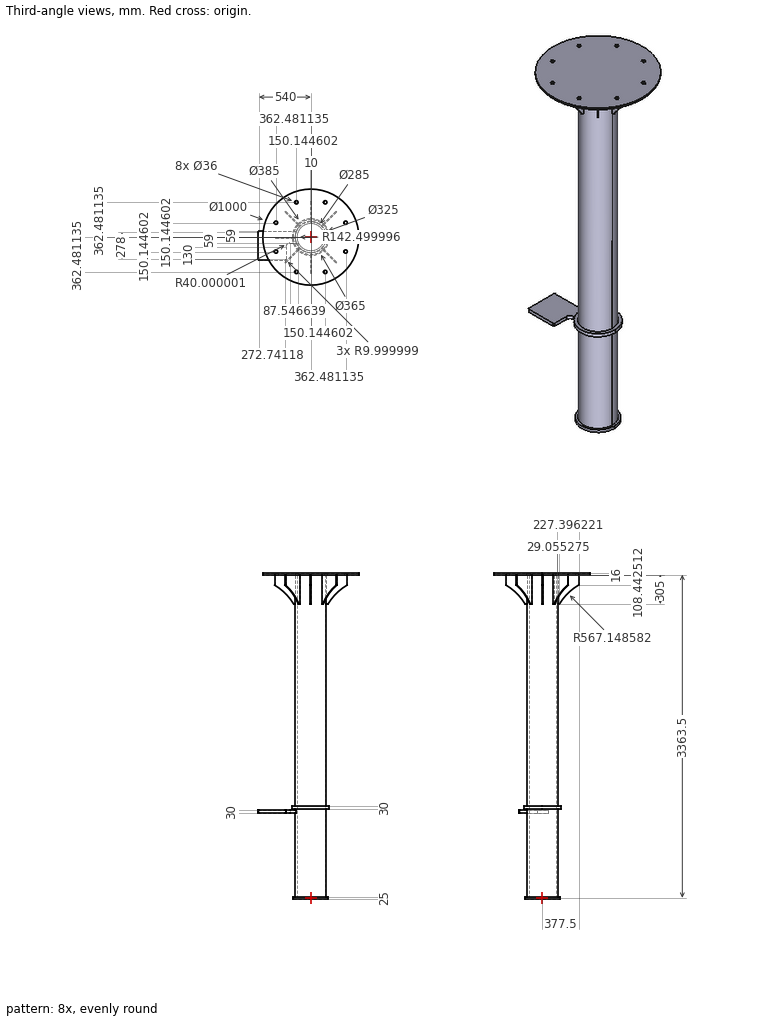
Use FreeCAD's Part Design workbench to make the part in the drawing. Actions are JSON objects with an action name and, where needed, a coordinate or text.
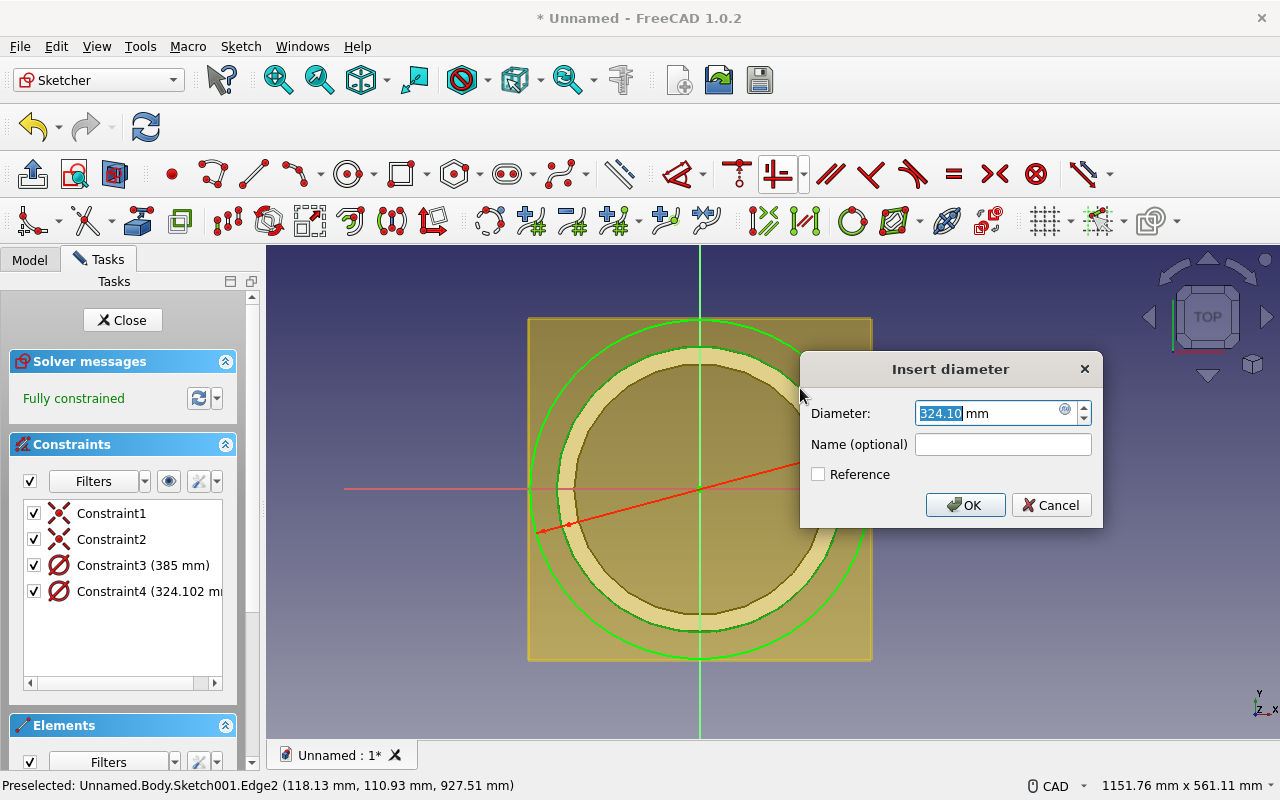
{"action": "type", "text": "325"}
{"action": "key", "text": "Return"}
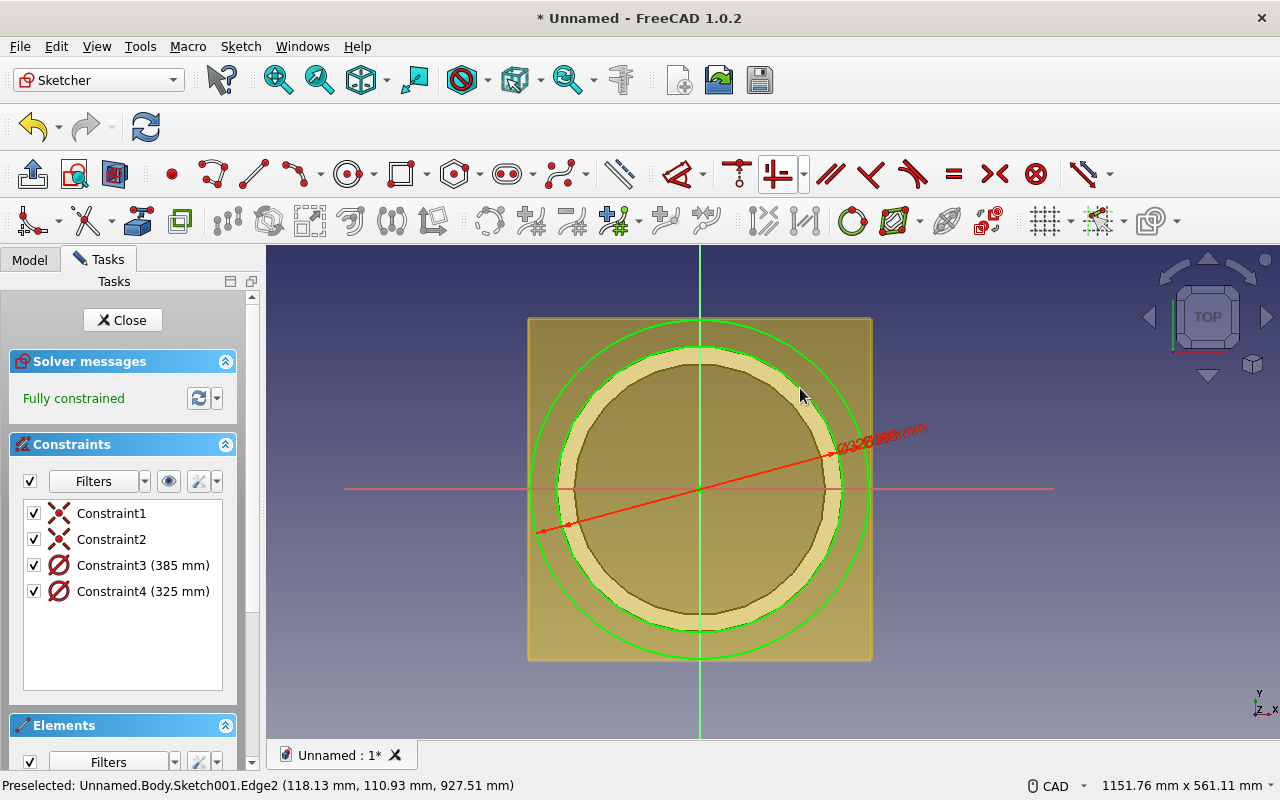
{"action": "left_click", "coordinate": [123, 320]}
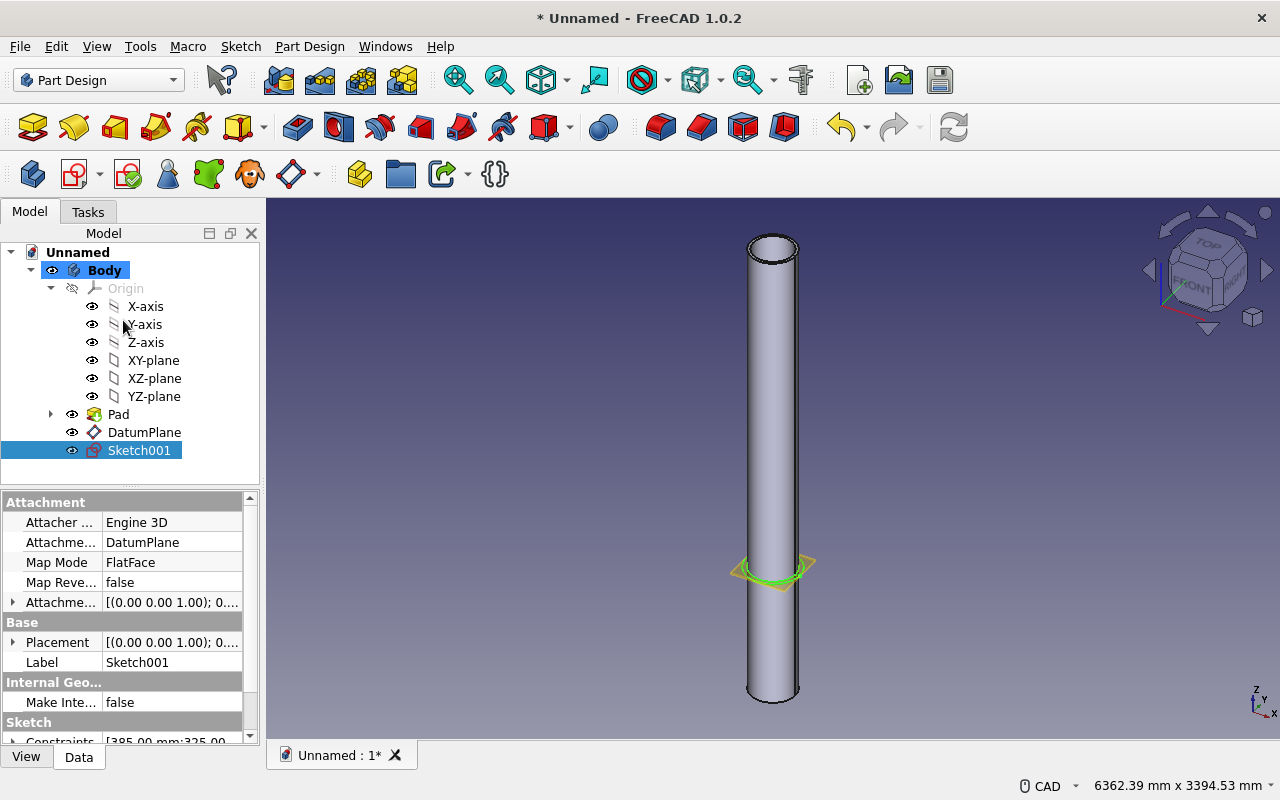
{"action": "left_click", "coordinate": [33, 128]}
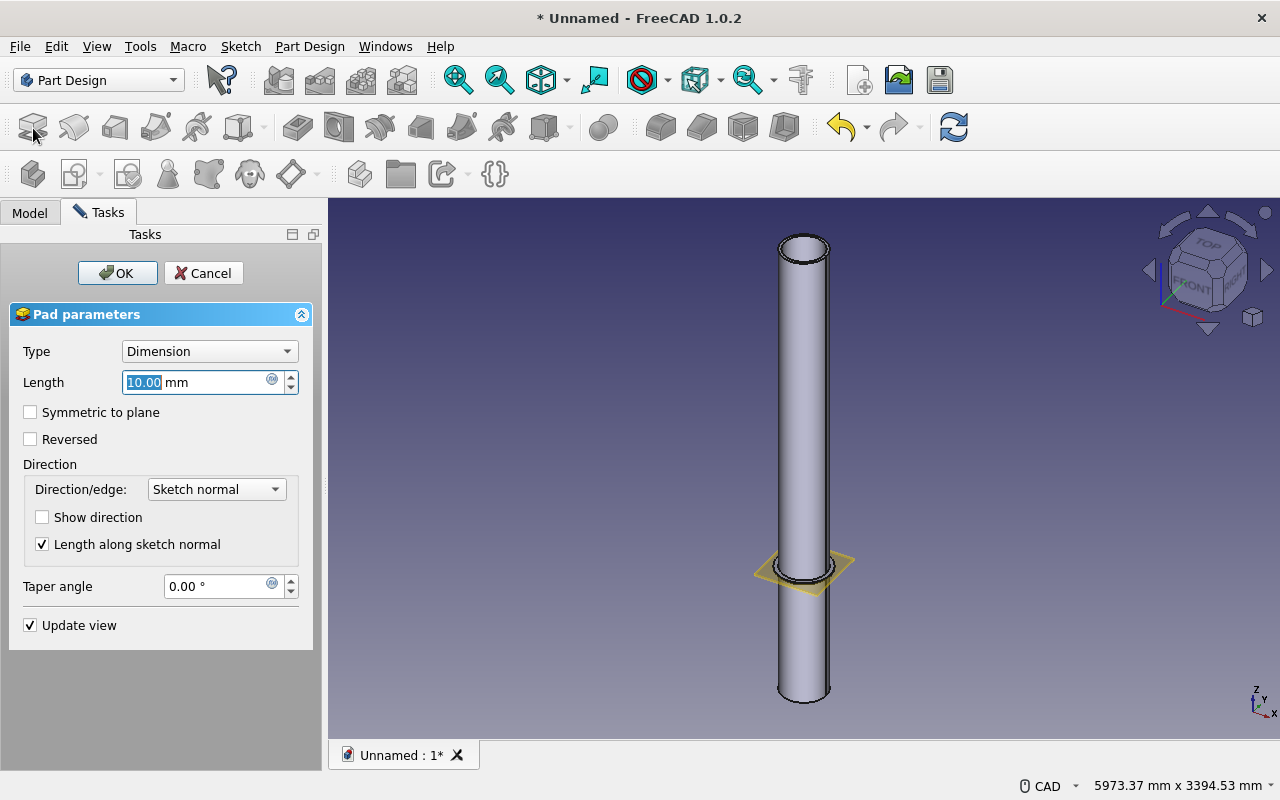
{"action": "type", "text": "30"}
{"action": "key", "text": "Tab"}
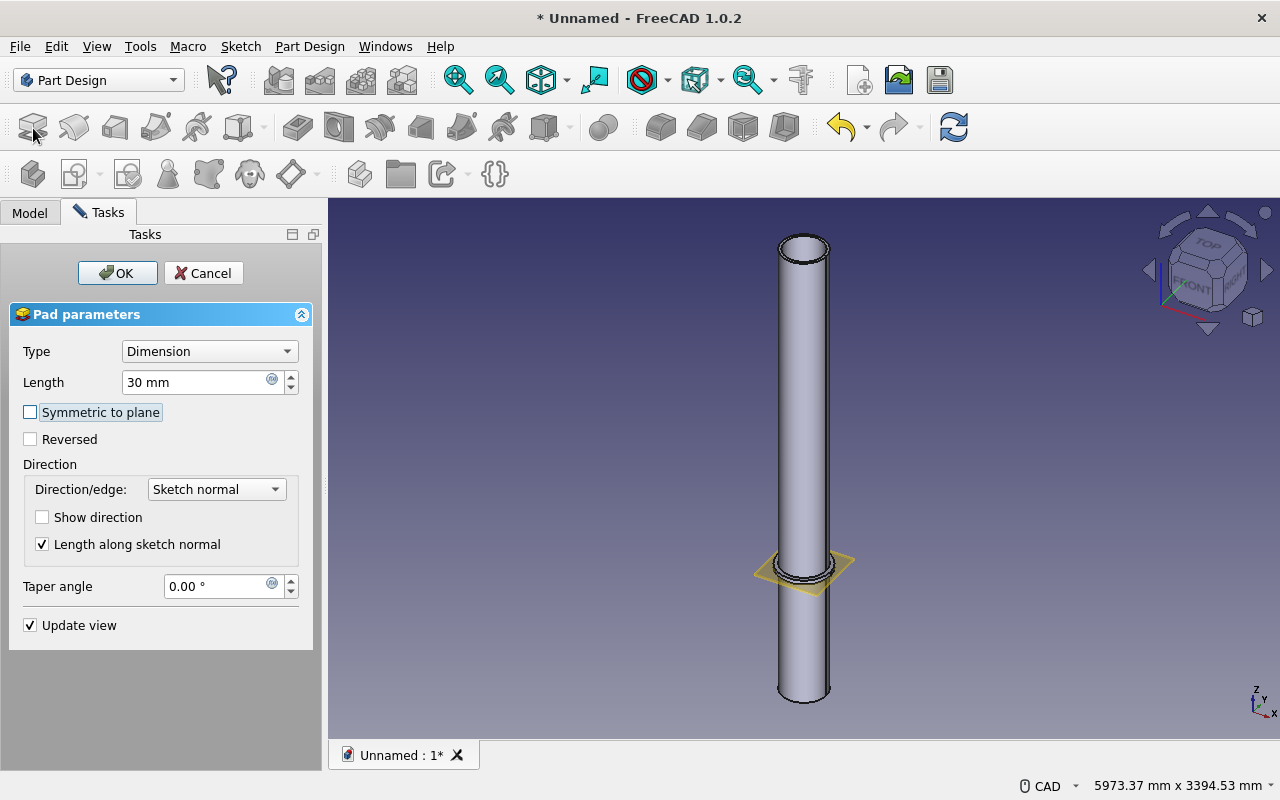
{"action": "left_click", "coordinate": [118, 273]}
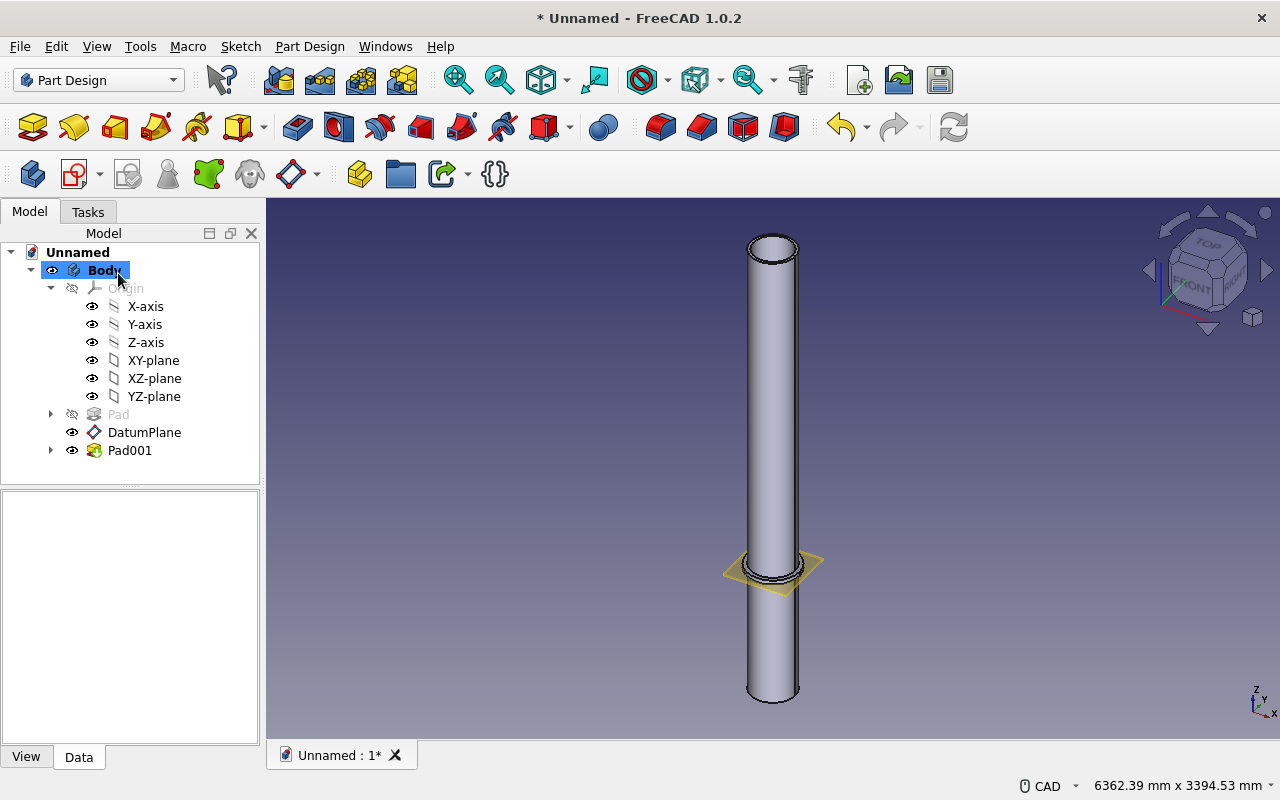
{"action": "left_click", "coordinate": [117, 432]}
{"action": "key", "text": "space"}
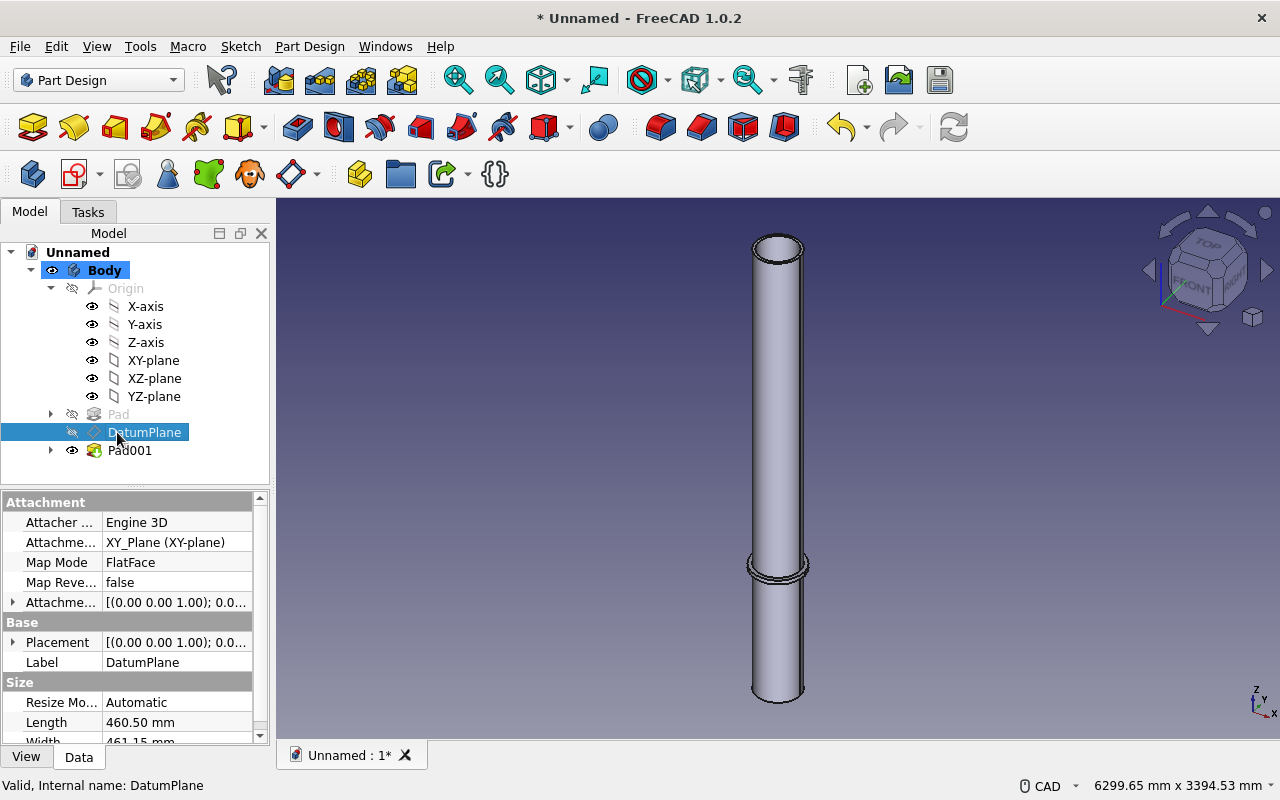
{"action": "scroll", "coordinate": [801, 251], "scroll_direction": "up", "scroll_amount": 15}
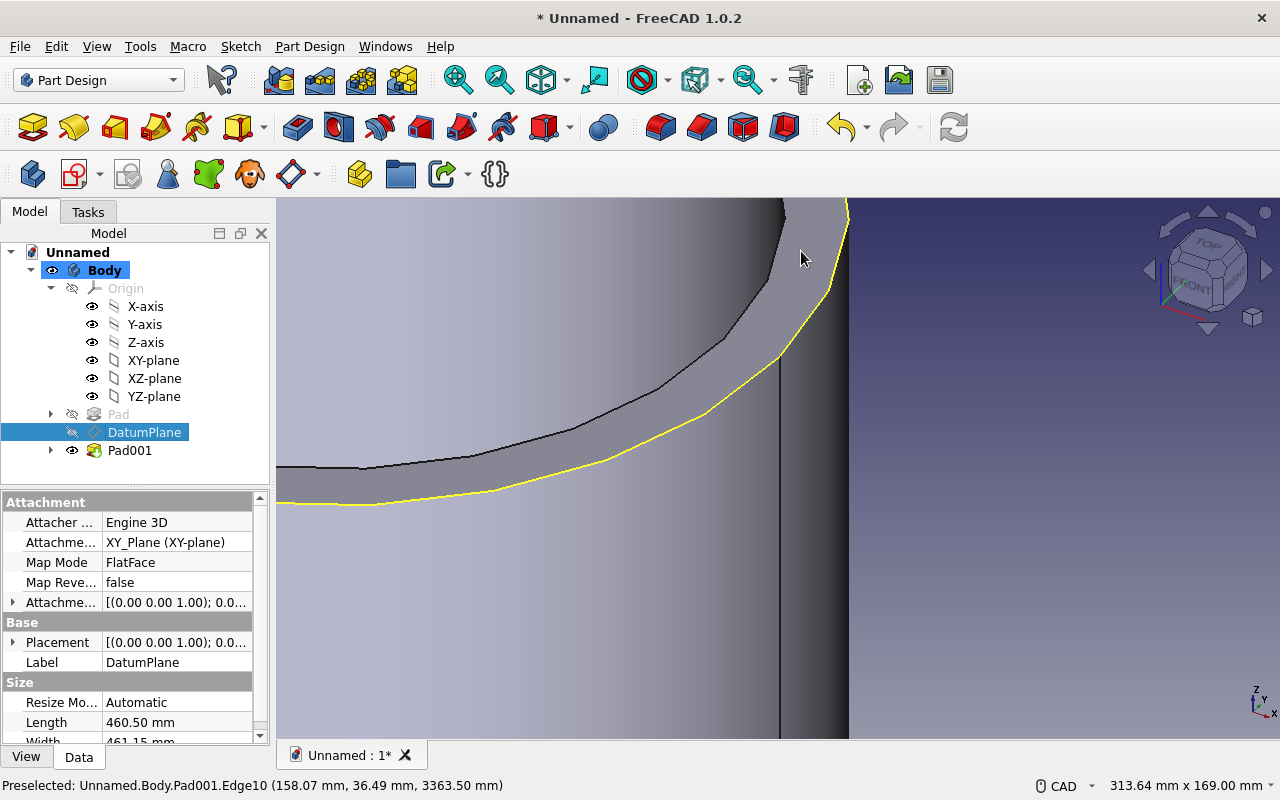
{"action": "left_click", "coordinate": [790, 261]}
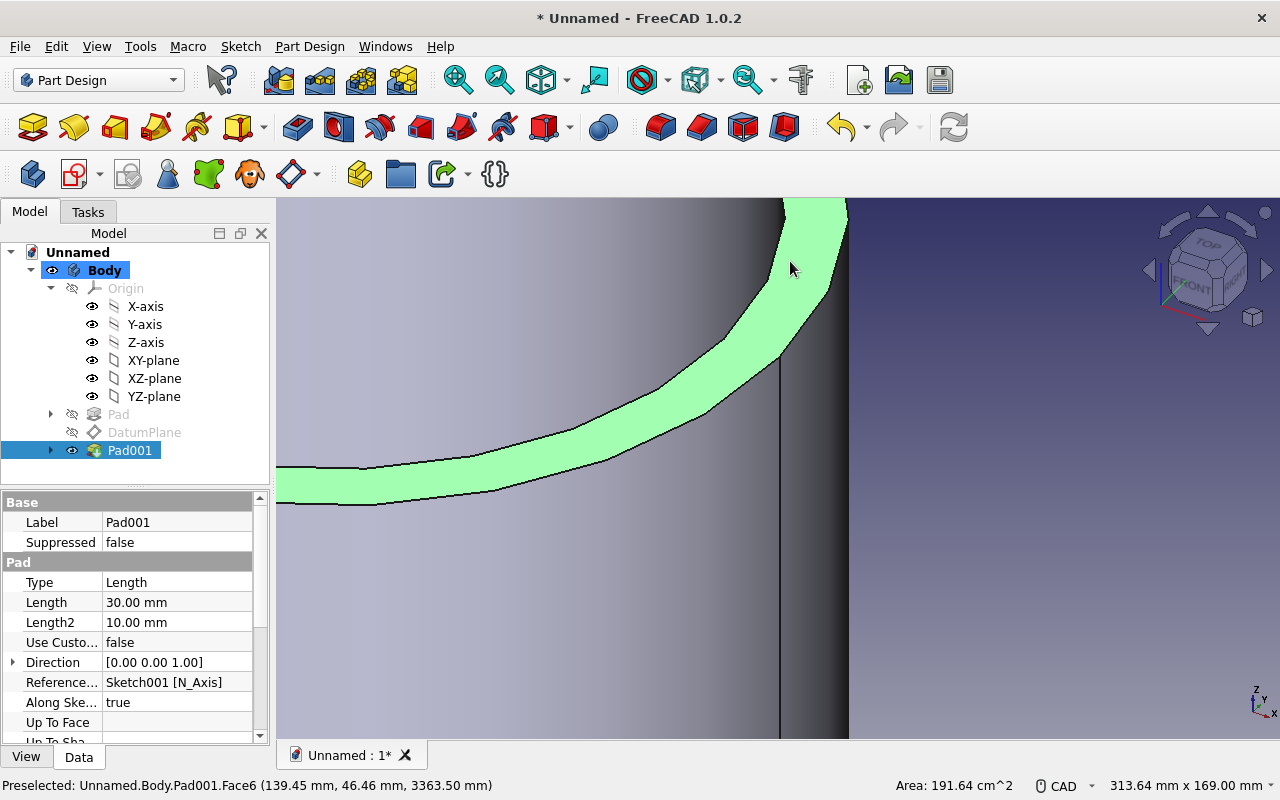
{"action": "left_click", "coordinate": [74, 174]}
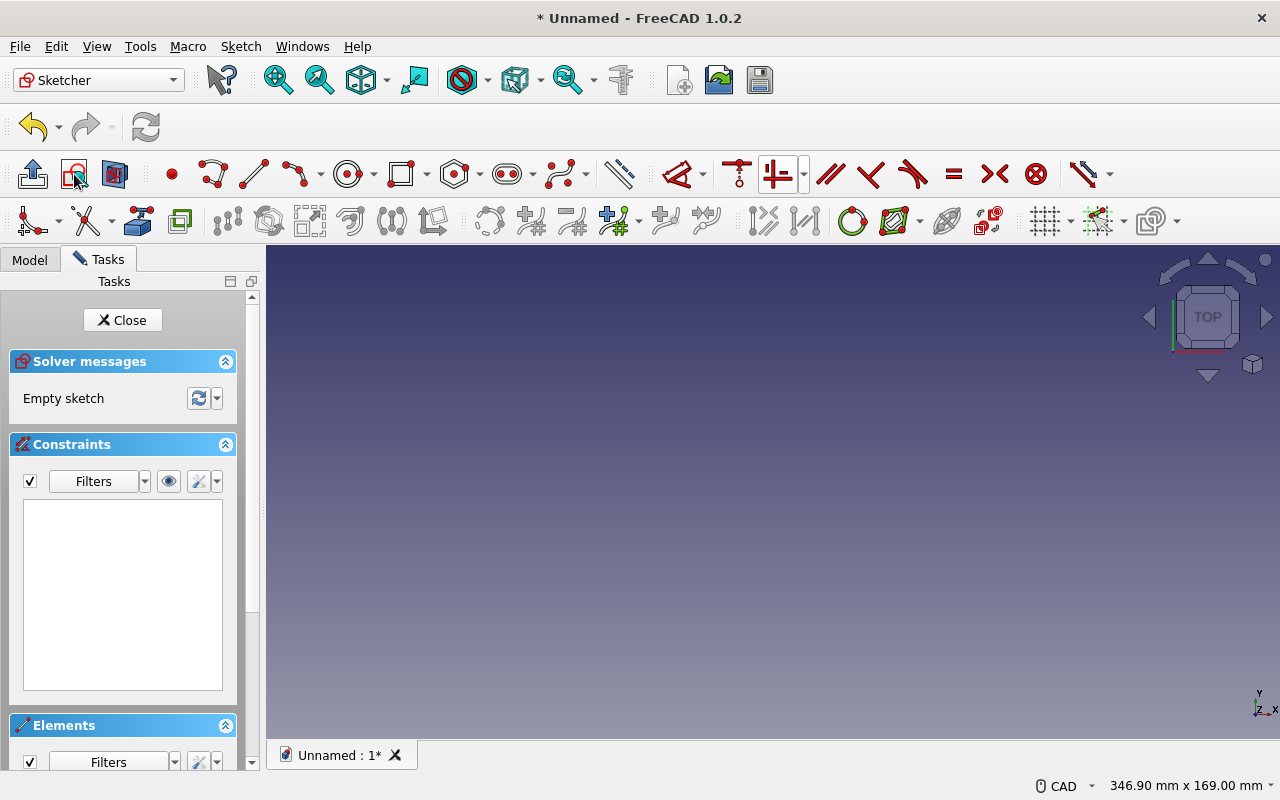
{"action": "scroll", "coordinate": [625, 284], "scroll_direction": "down", "scroll_amount": 12}